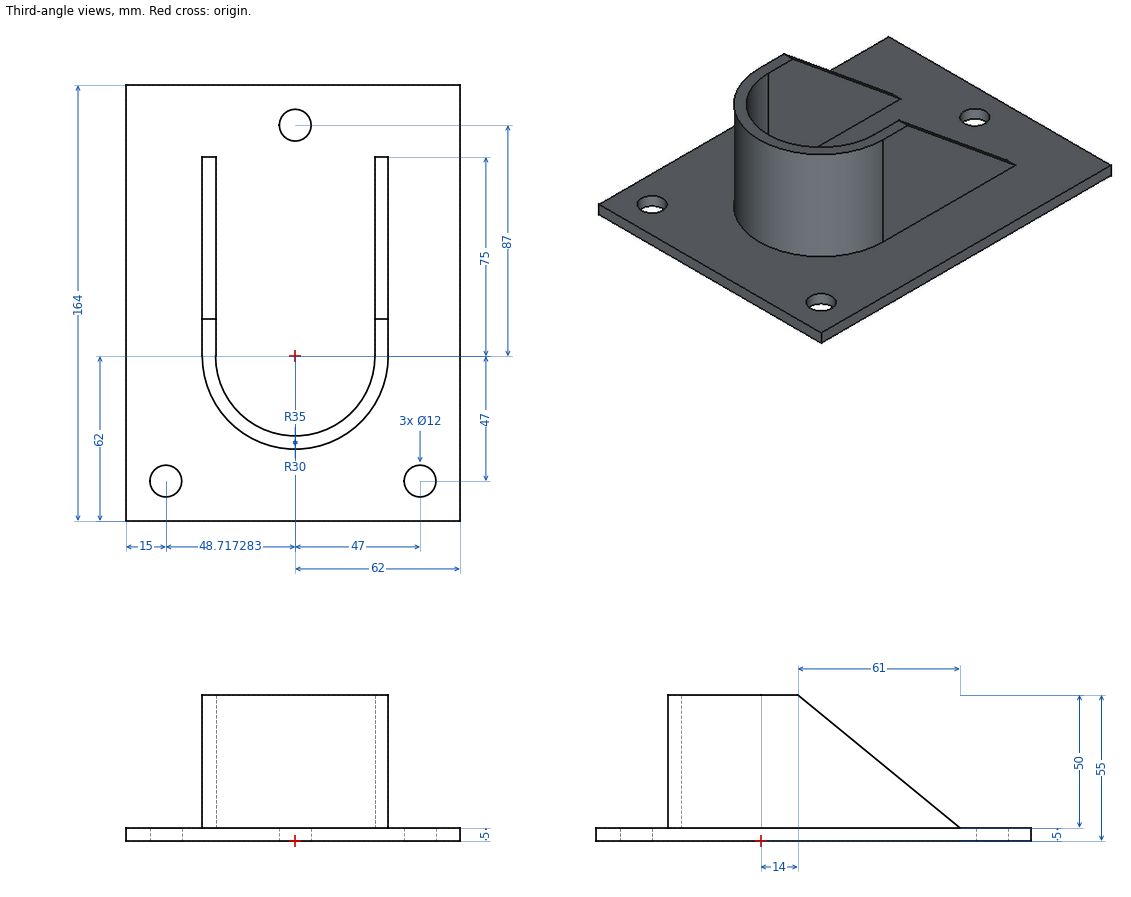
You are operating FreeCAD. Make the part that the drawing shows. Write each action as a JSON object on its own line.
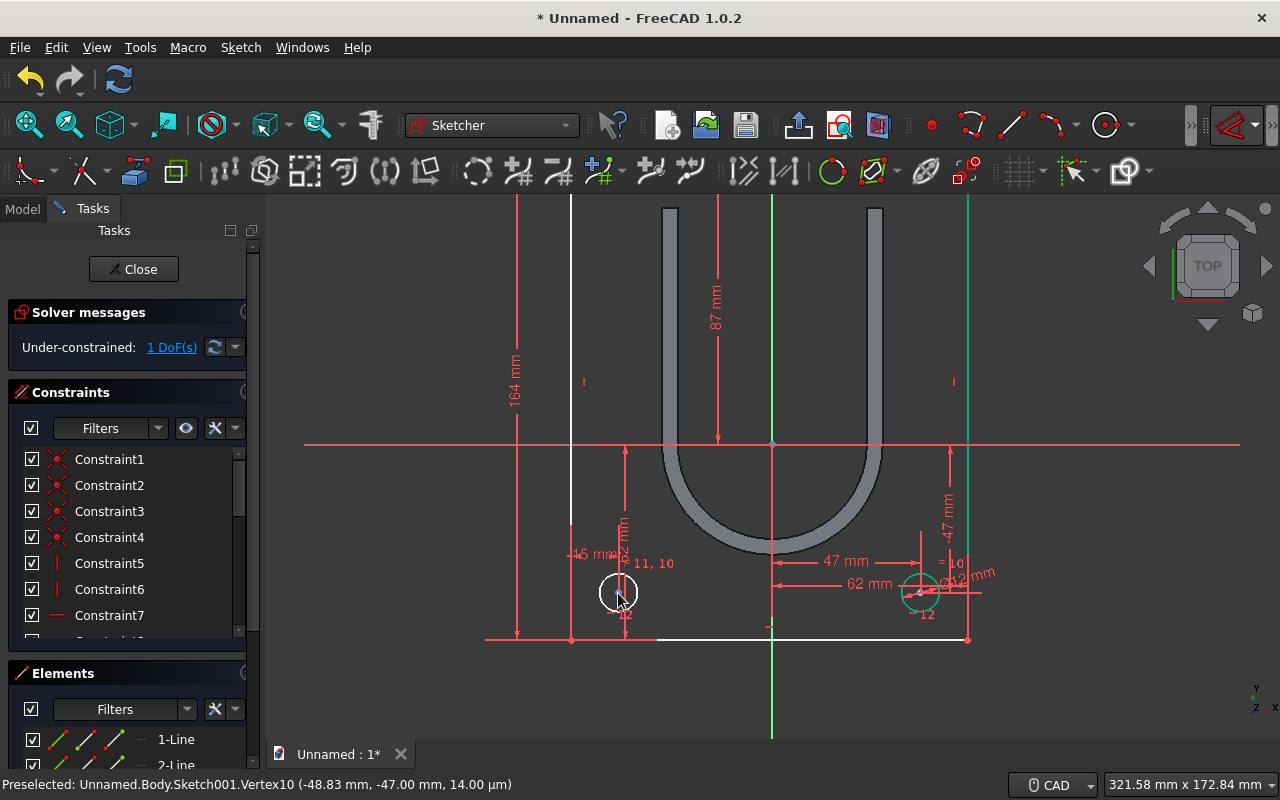
{"action": "left_click", "coordinate": [619, 593]}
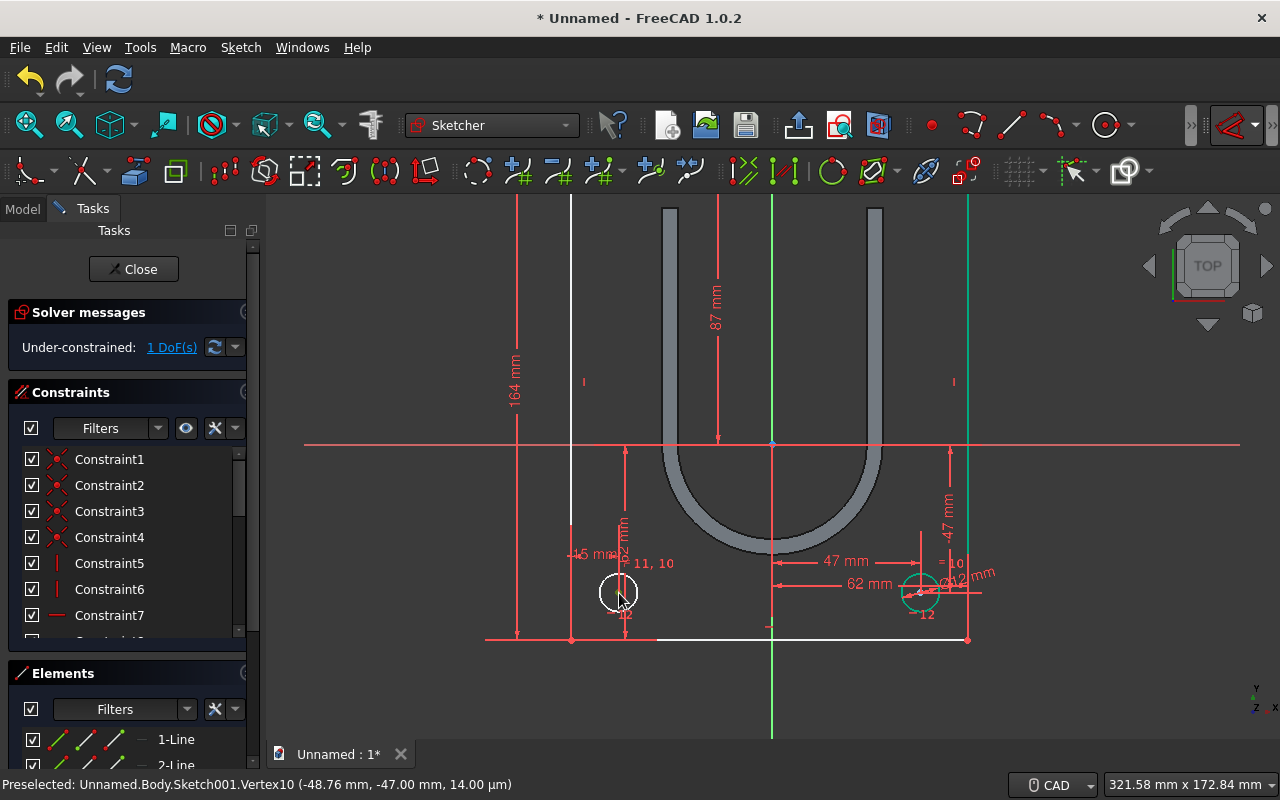
{"action": "left_click", "coordinate": [1258, 126]}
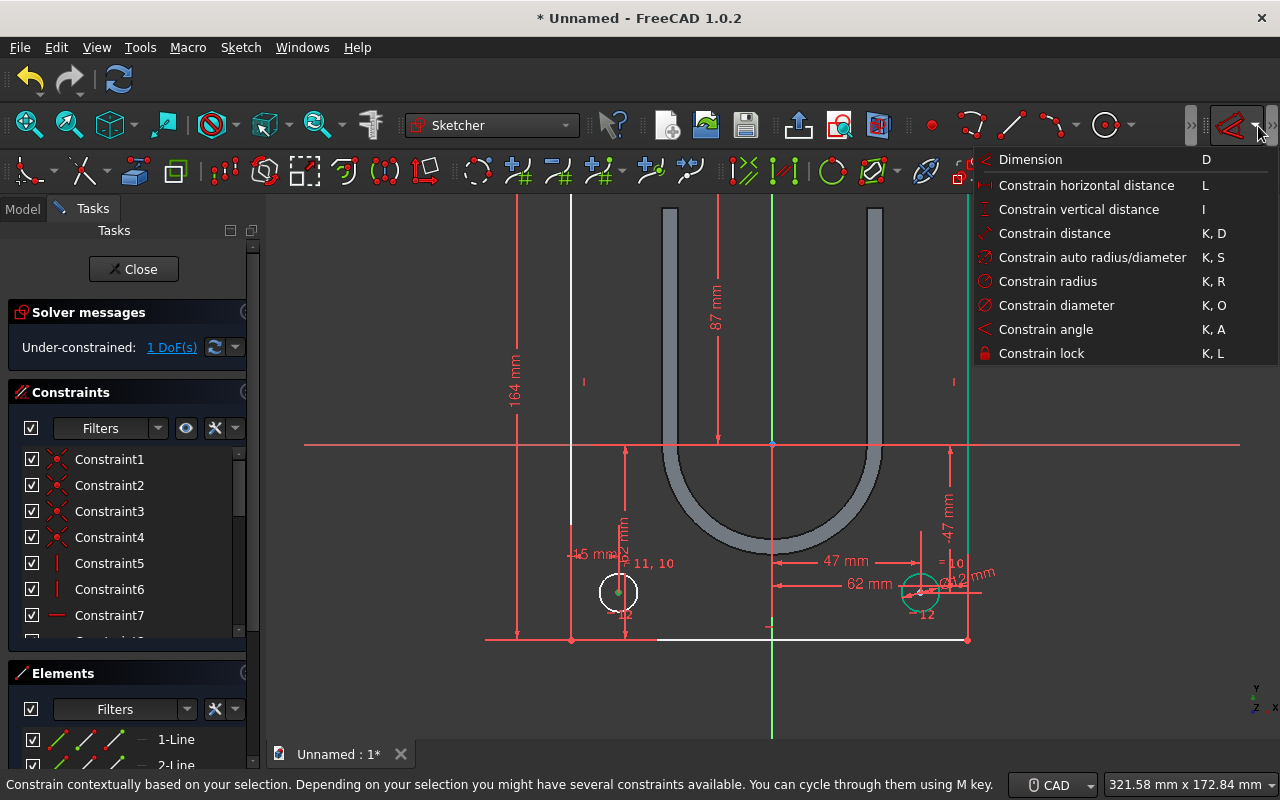
{"action": "left_click", "coordinate": [1126, 185]}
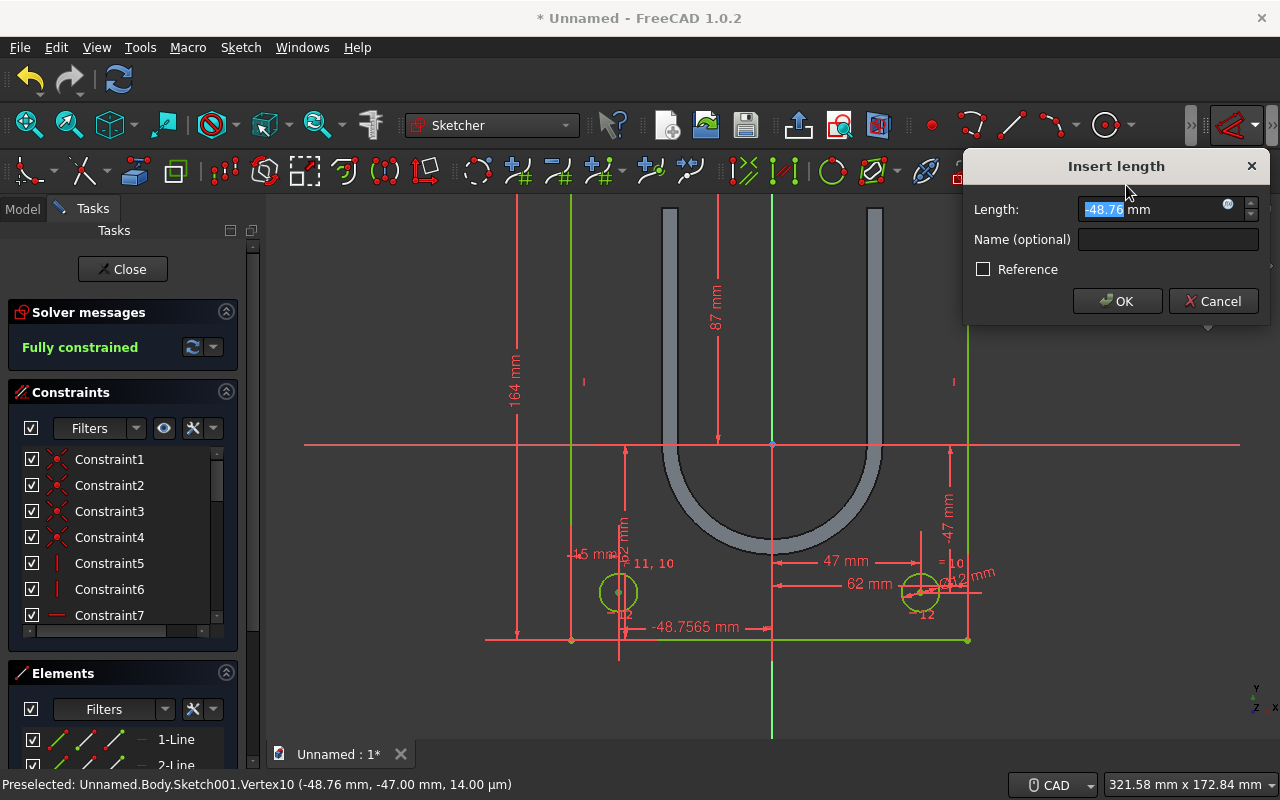
{"action": "type", "text": "-48.717283"}
{"action": "key", "text": "Return"}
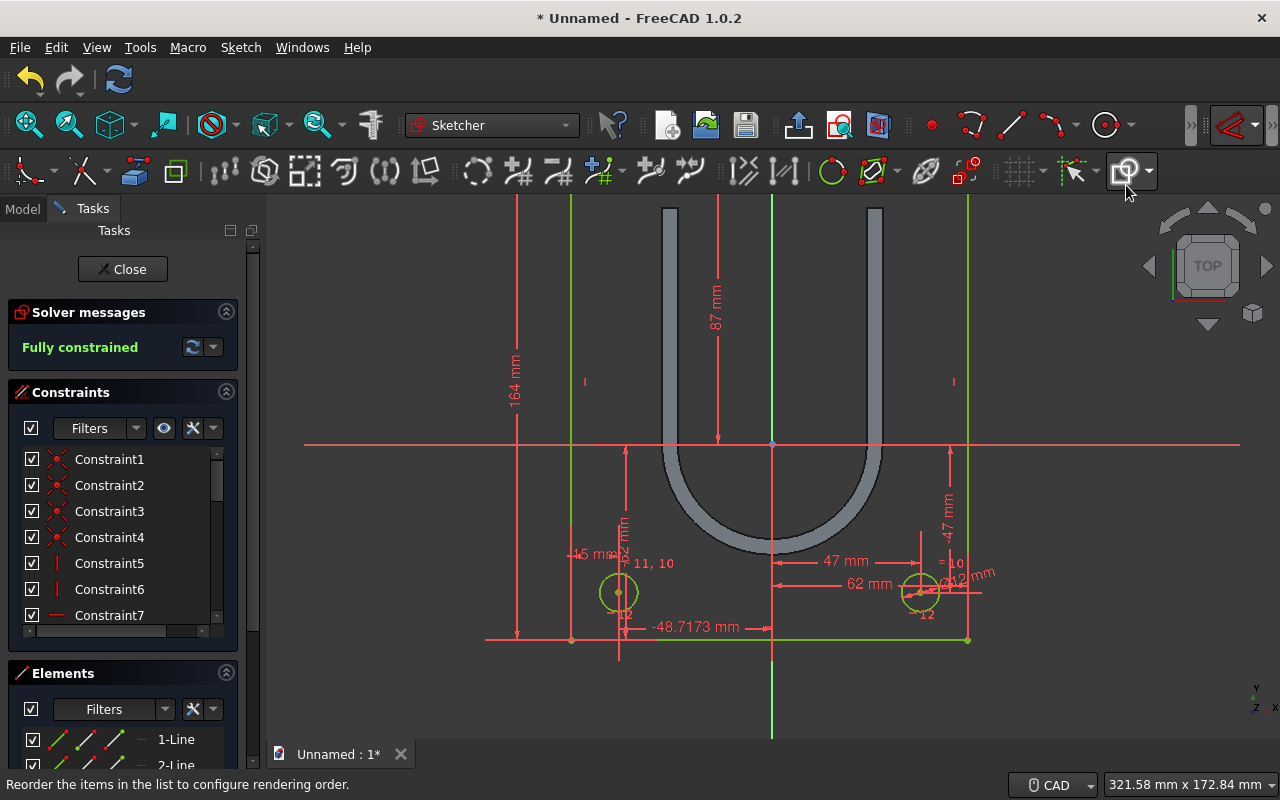
{"action": "left_click", "coordinate": [123, 269]}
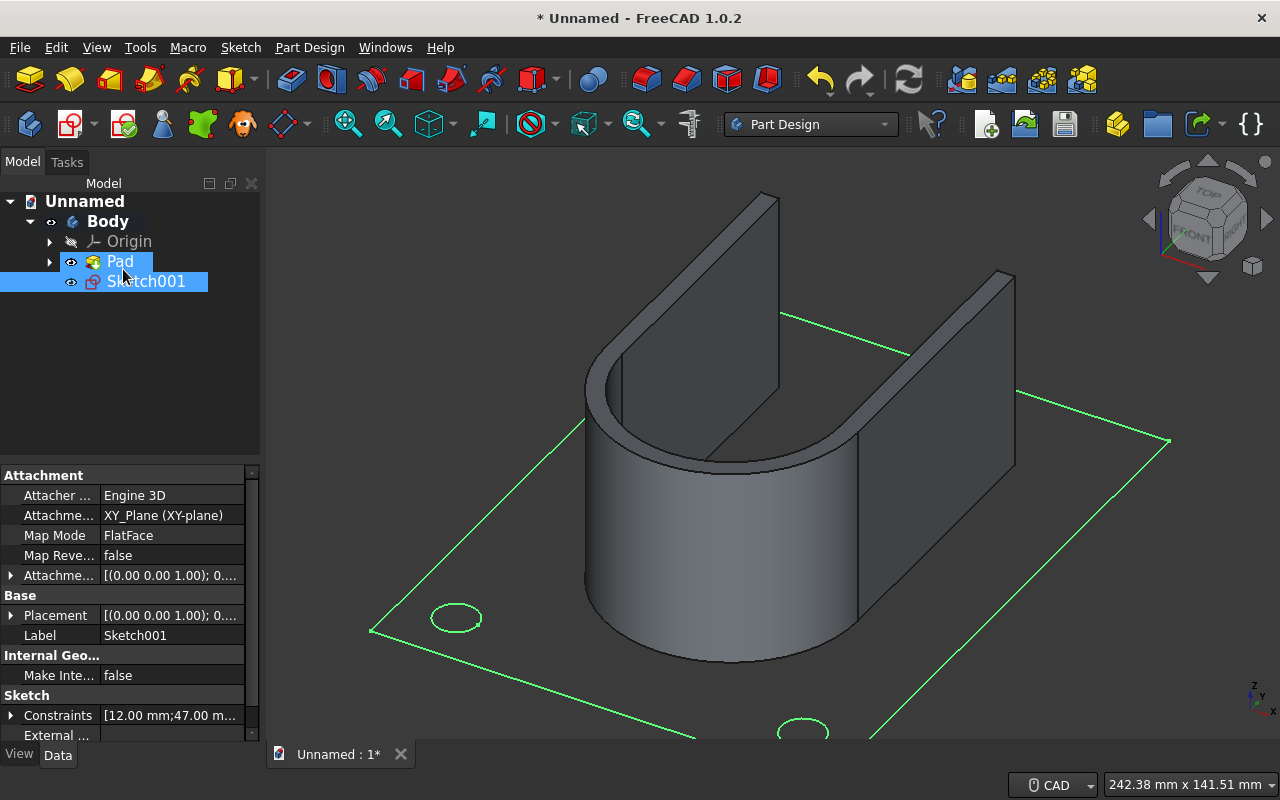
{"action": "left_click", "coordinate": [30, 80]}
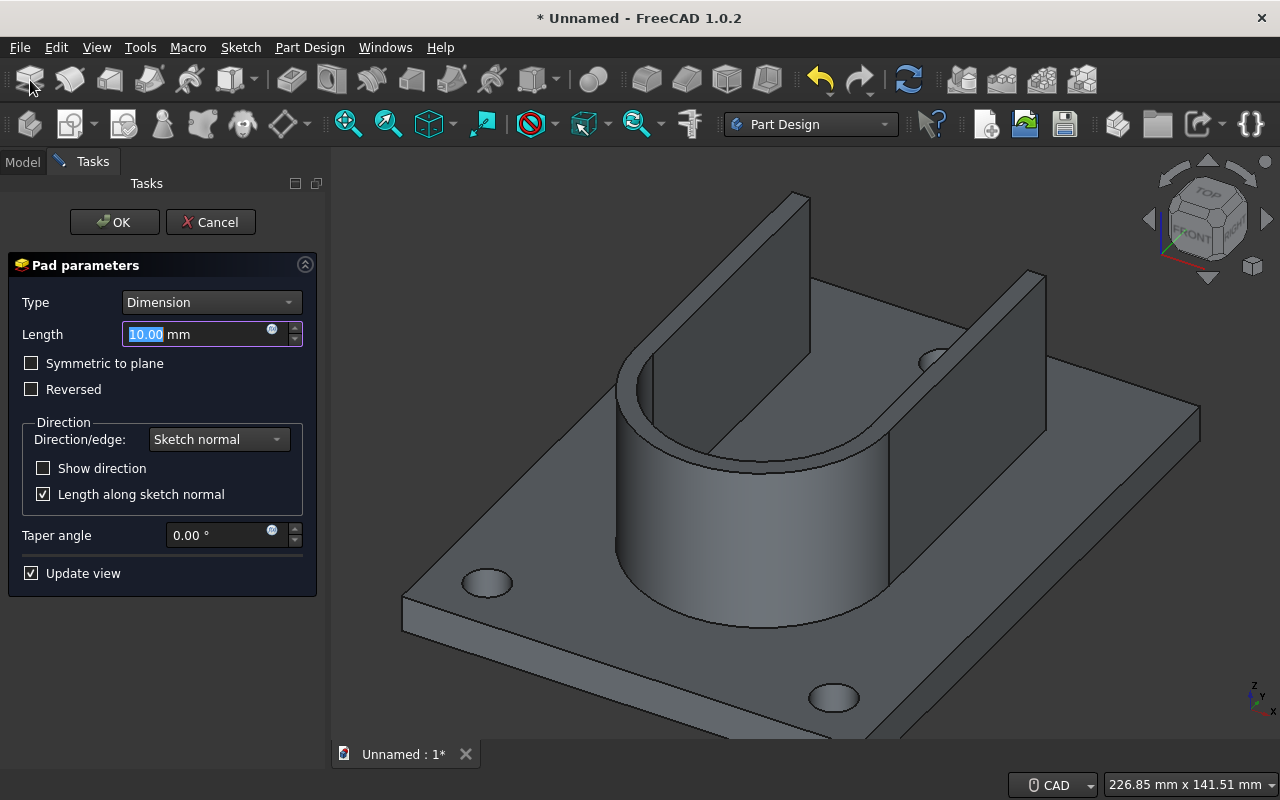
{"action": "type", "text": "5"}
{"action": "key", "text": "Tab"}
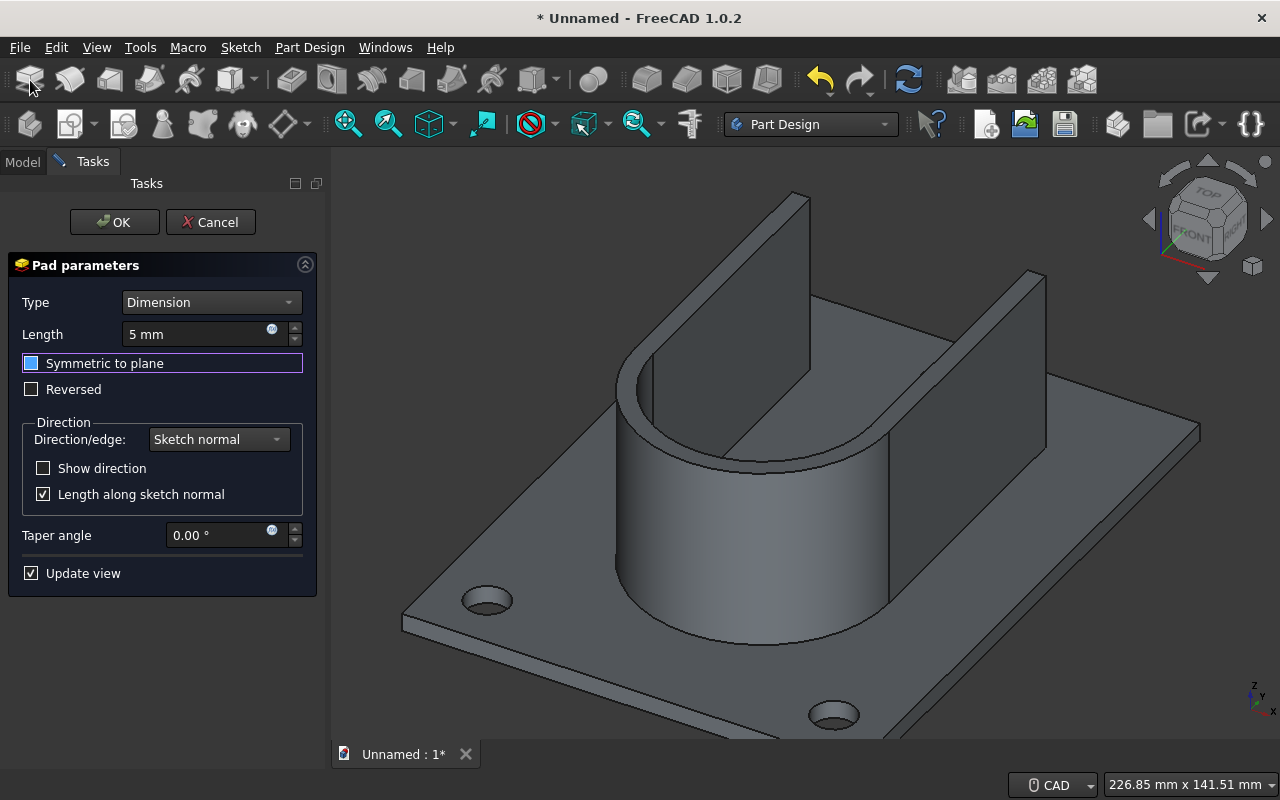
{"action": "left_click", "coordinate": [115, 222]}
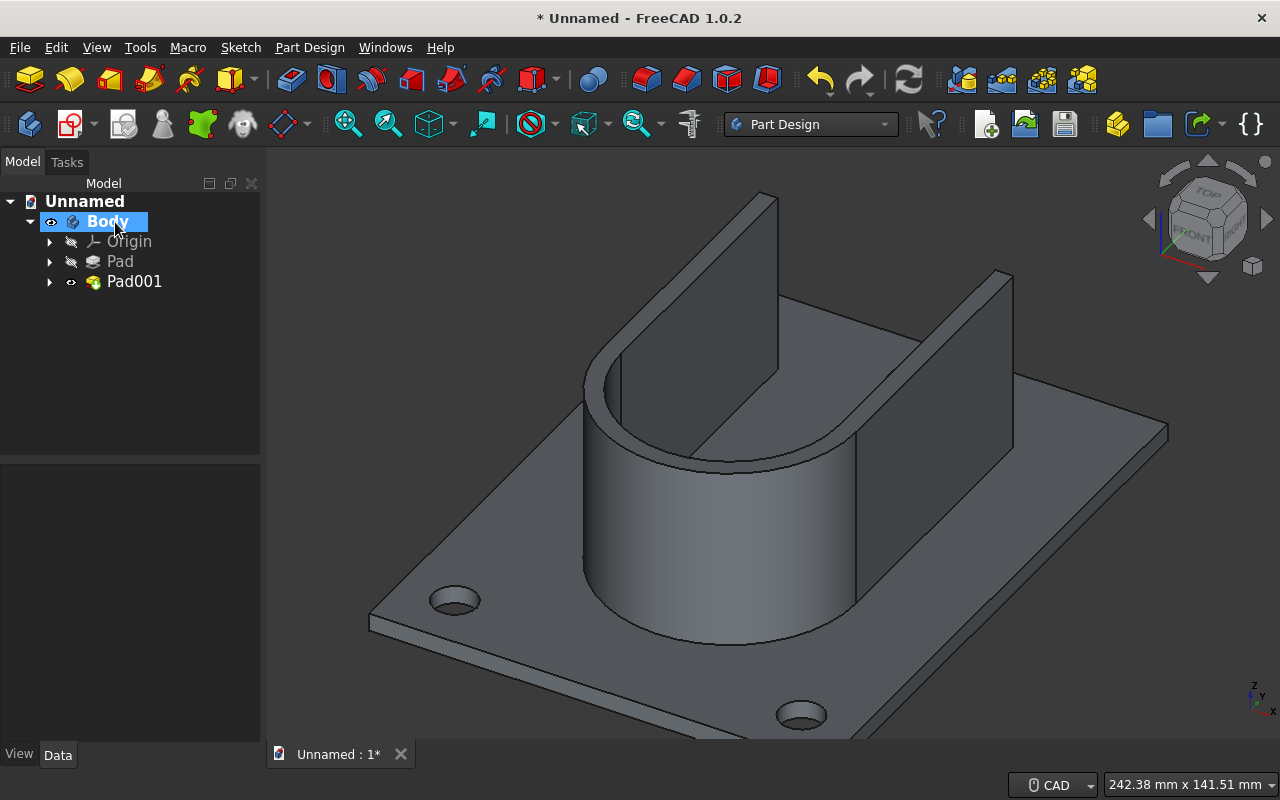
{"action": "left_click", "coordinate": [350, 124]}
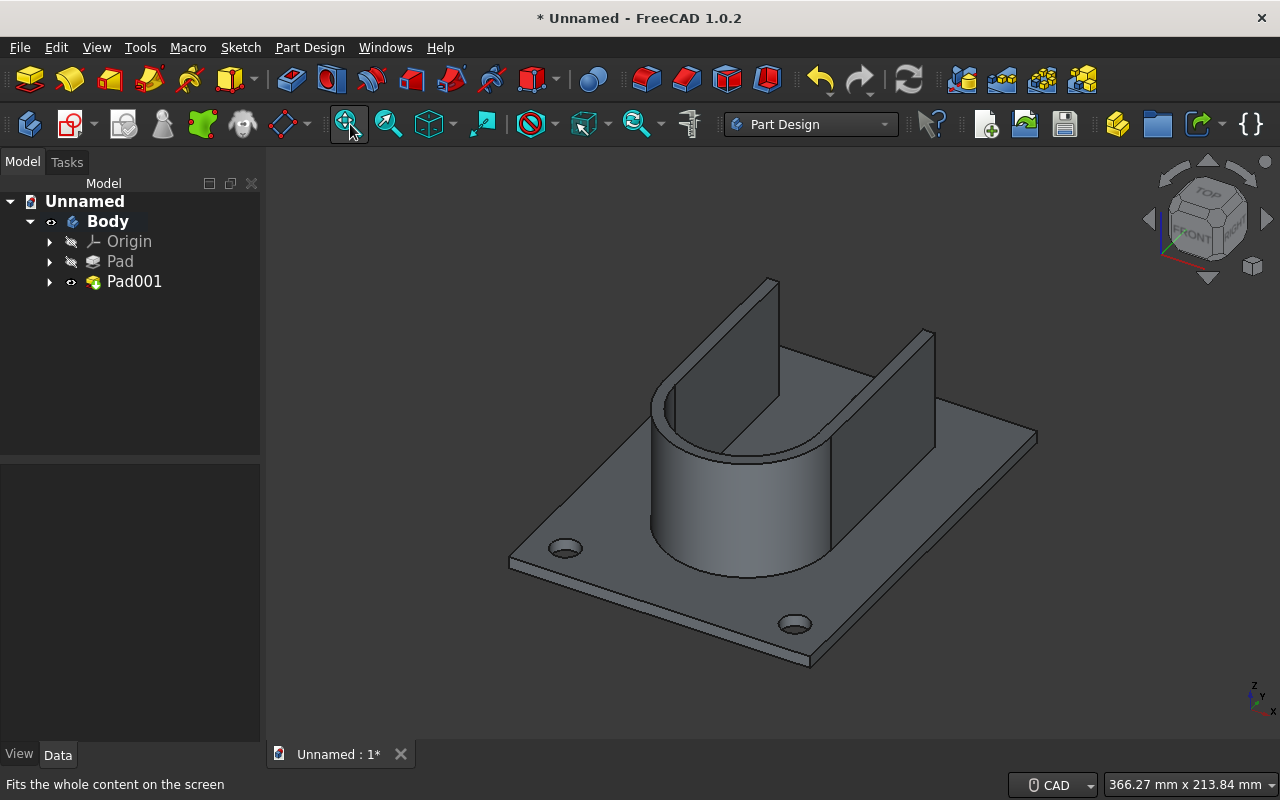
{"action": "scroll", "coordinate": [1021, 452], "scroll_direction": "up", "scroll_amount": 3}